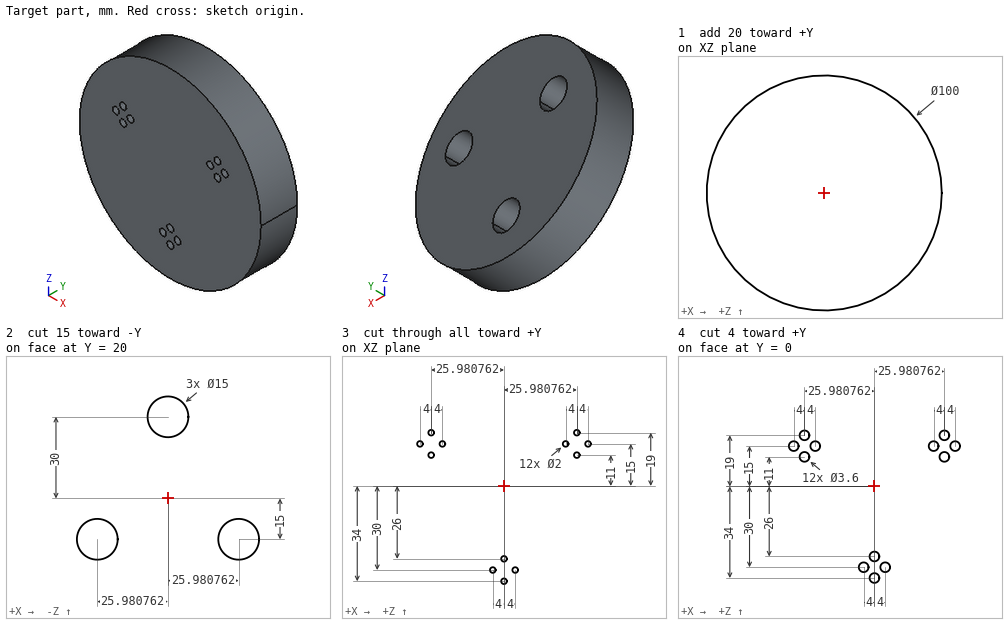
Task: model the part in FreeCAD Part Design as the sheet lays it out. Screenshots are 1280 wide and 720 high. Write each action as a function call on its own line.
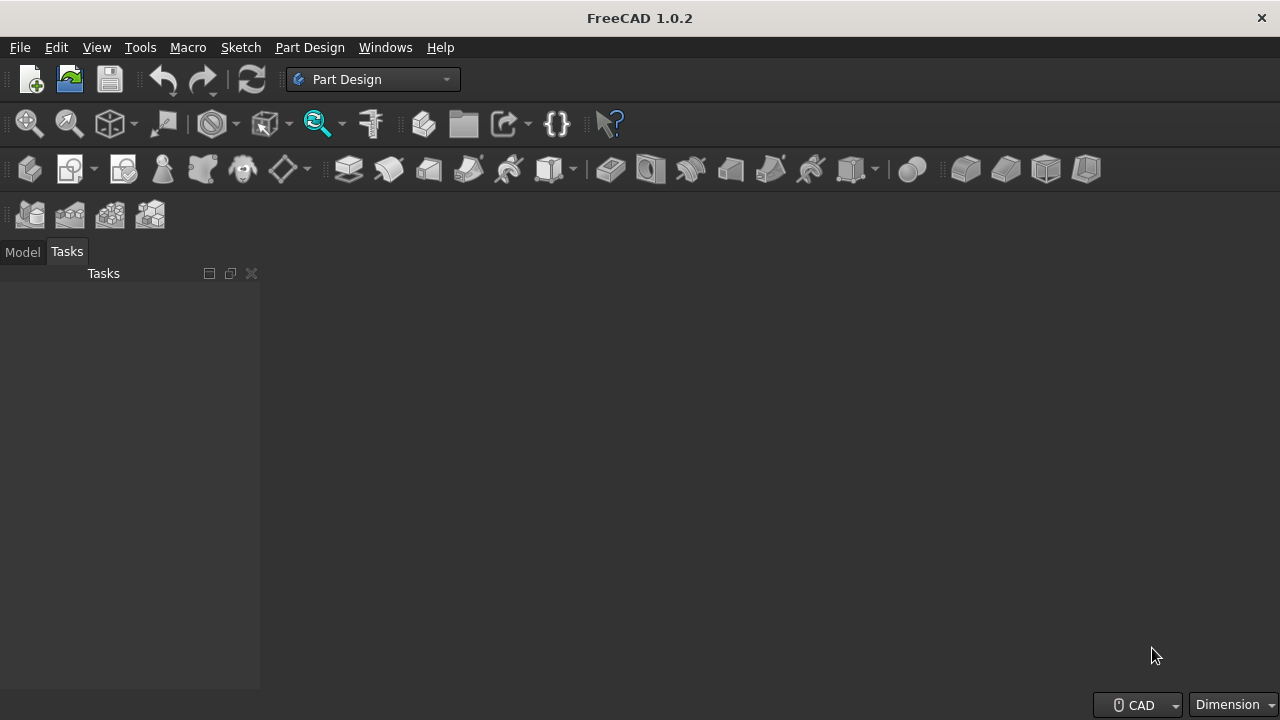
click(30, 80)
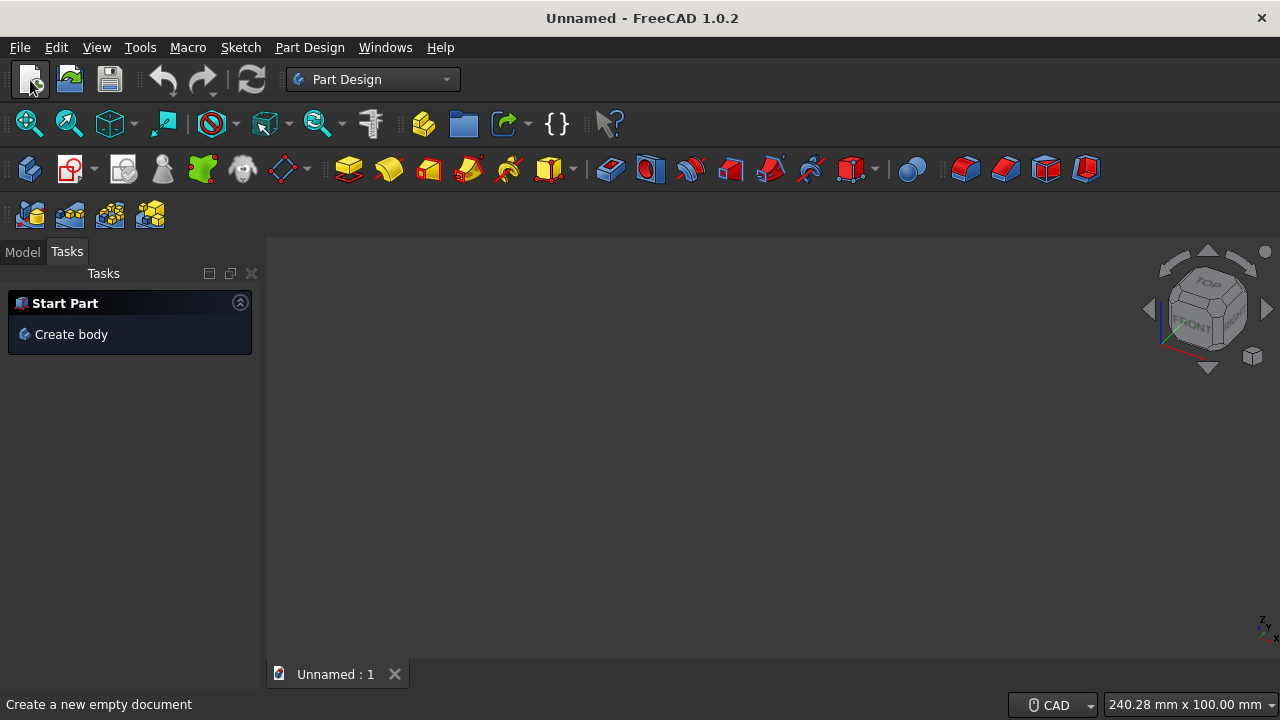
click(70, 170)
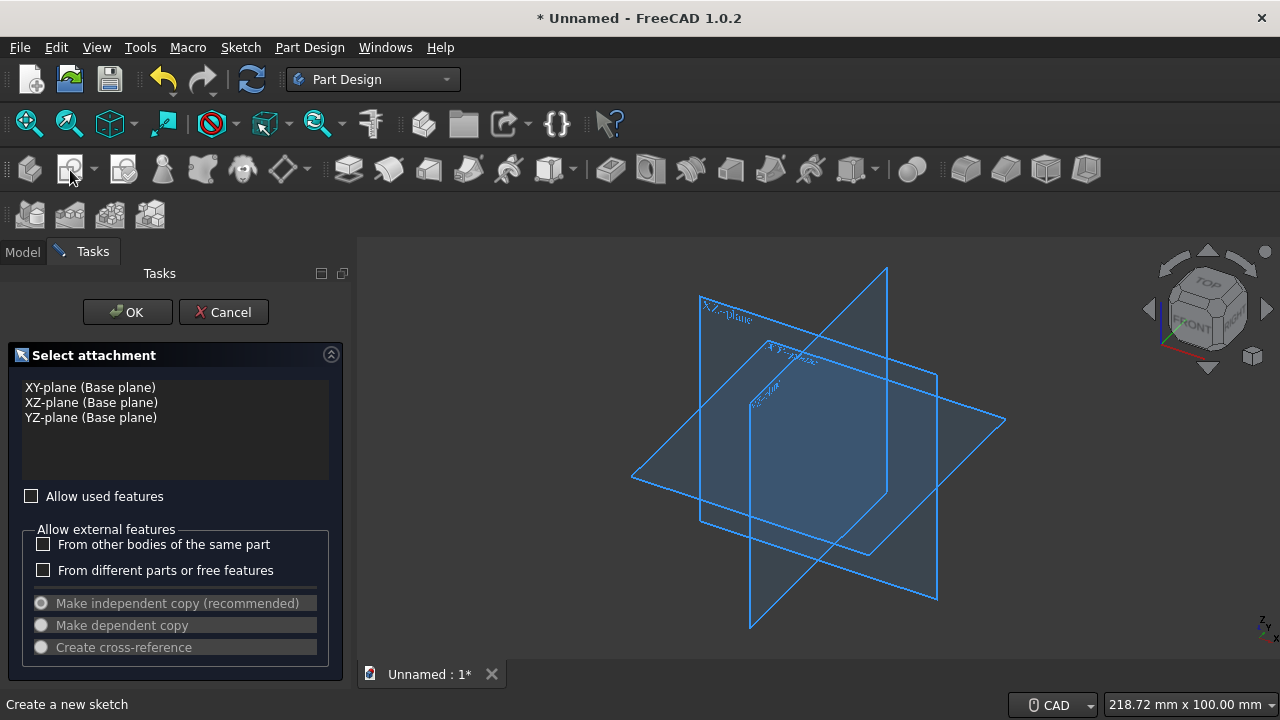
click(82, 402)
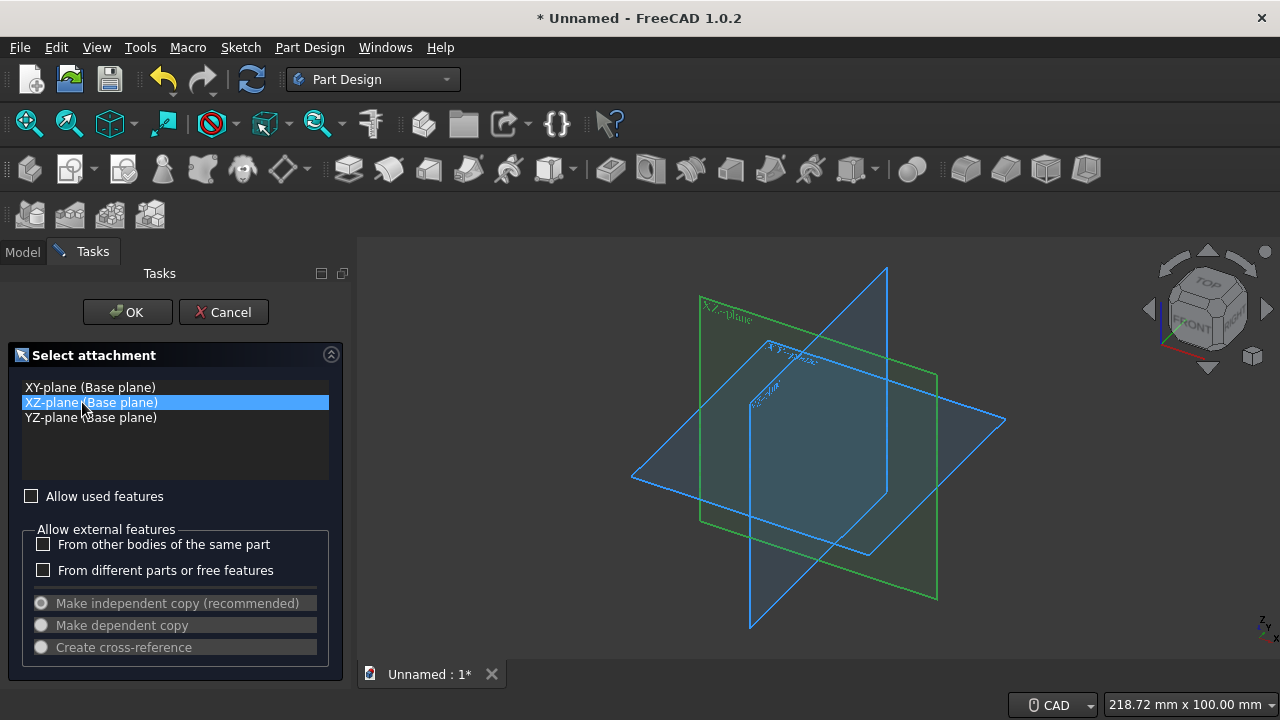
click(128, 312)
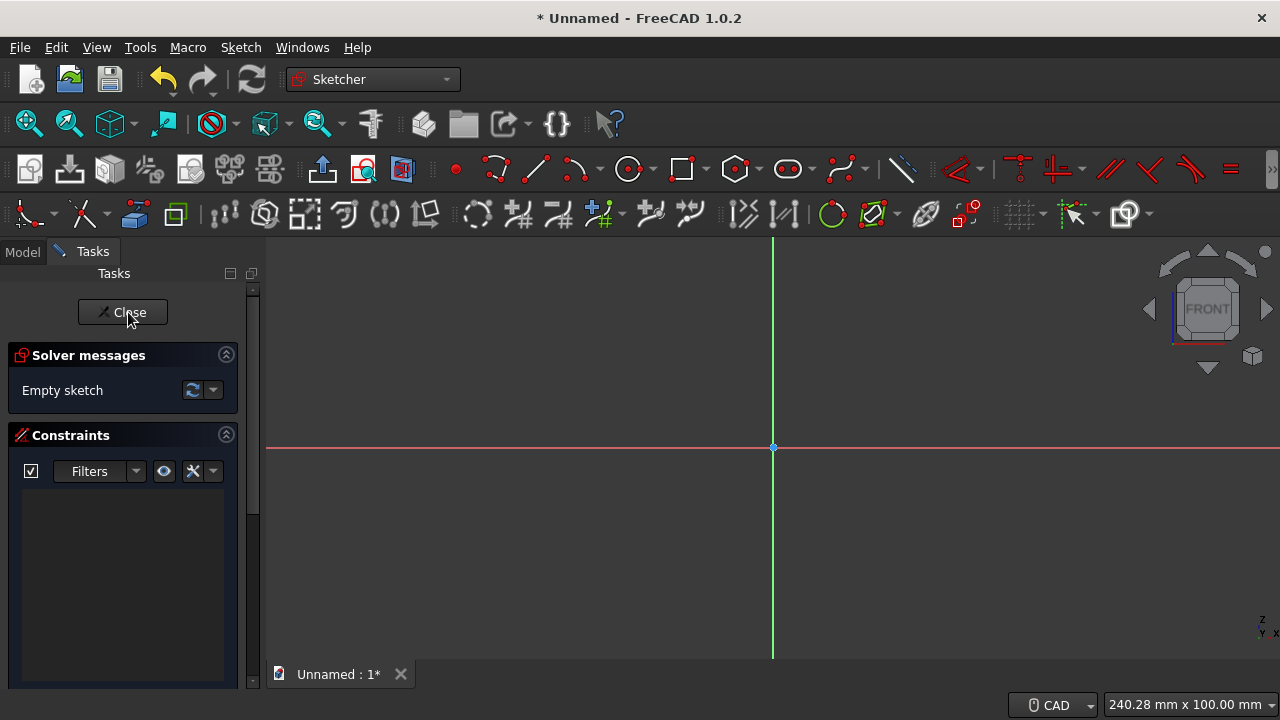
scroll(565, 448, down, 2)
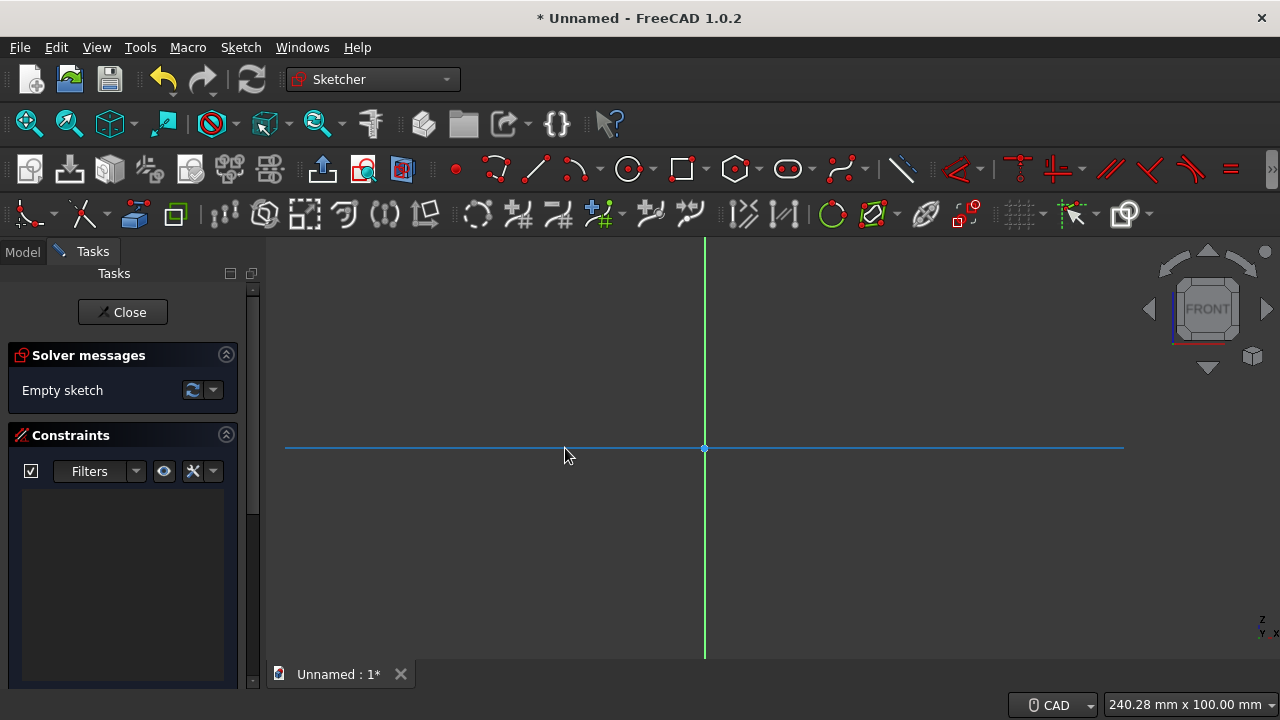
click(630, 170)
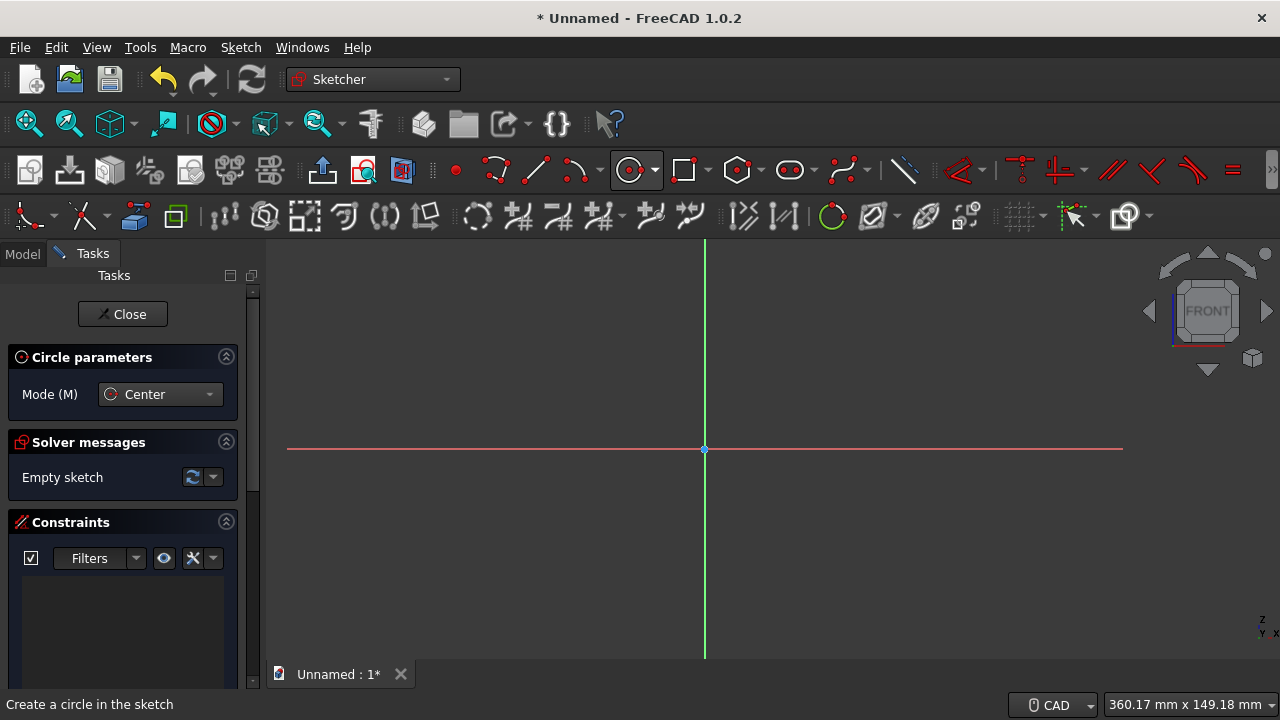
click(705, 449)
click(804, 350)
key(Escape)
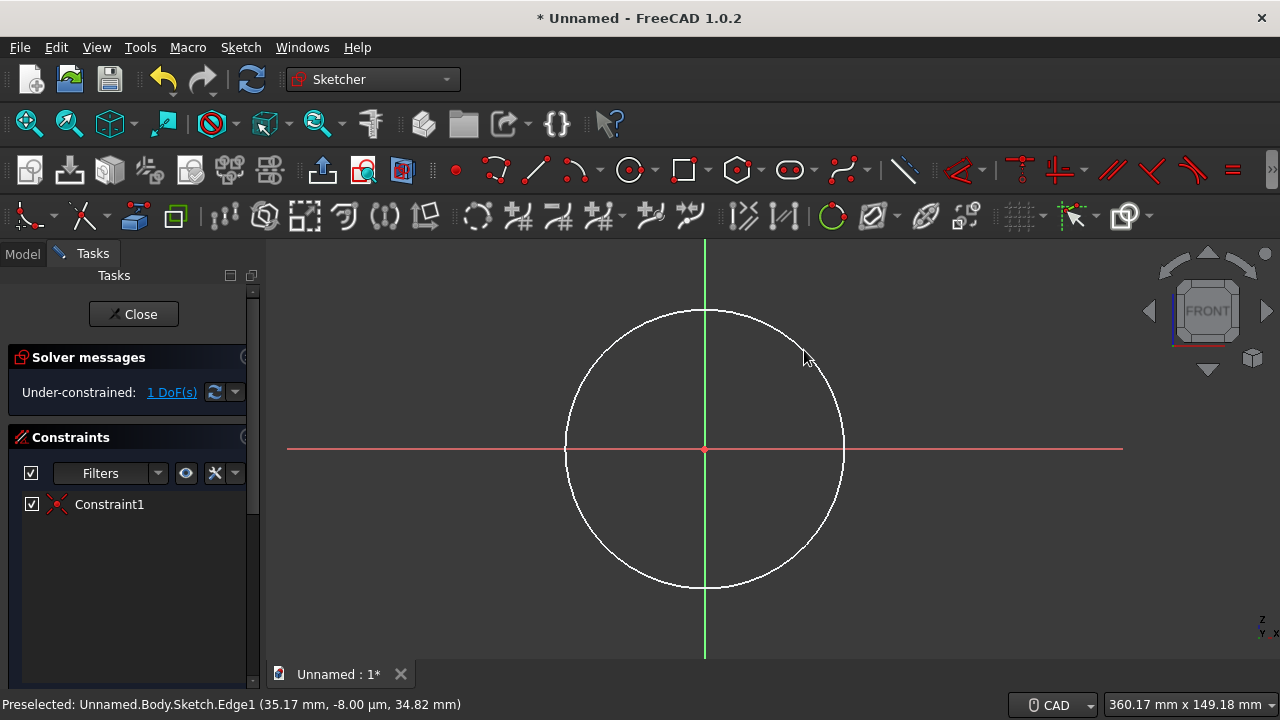
click(803, 350)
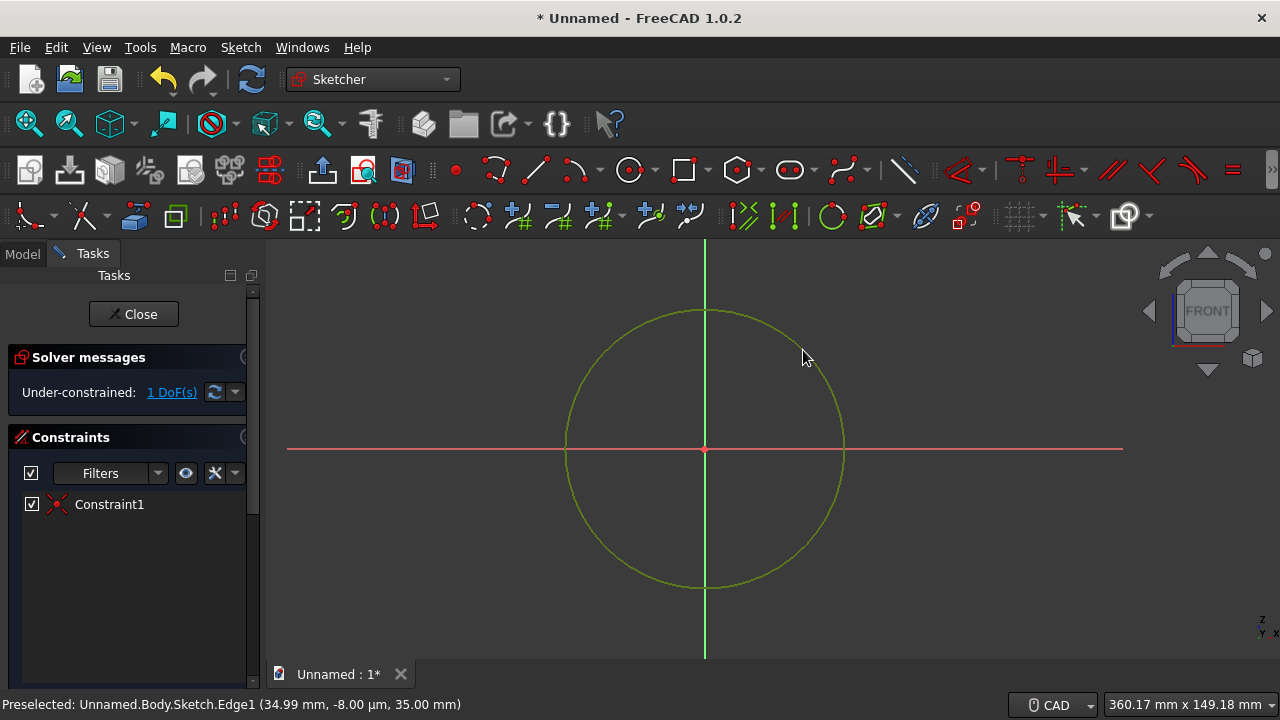
click(984, 170)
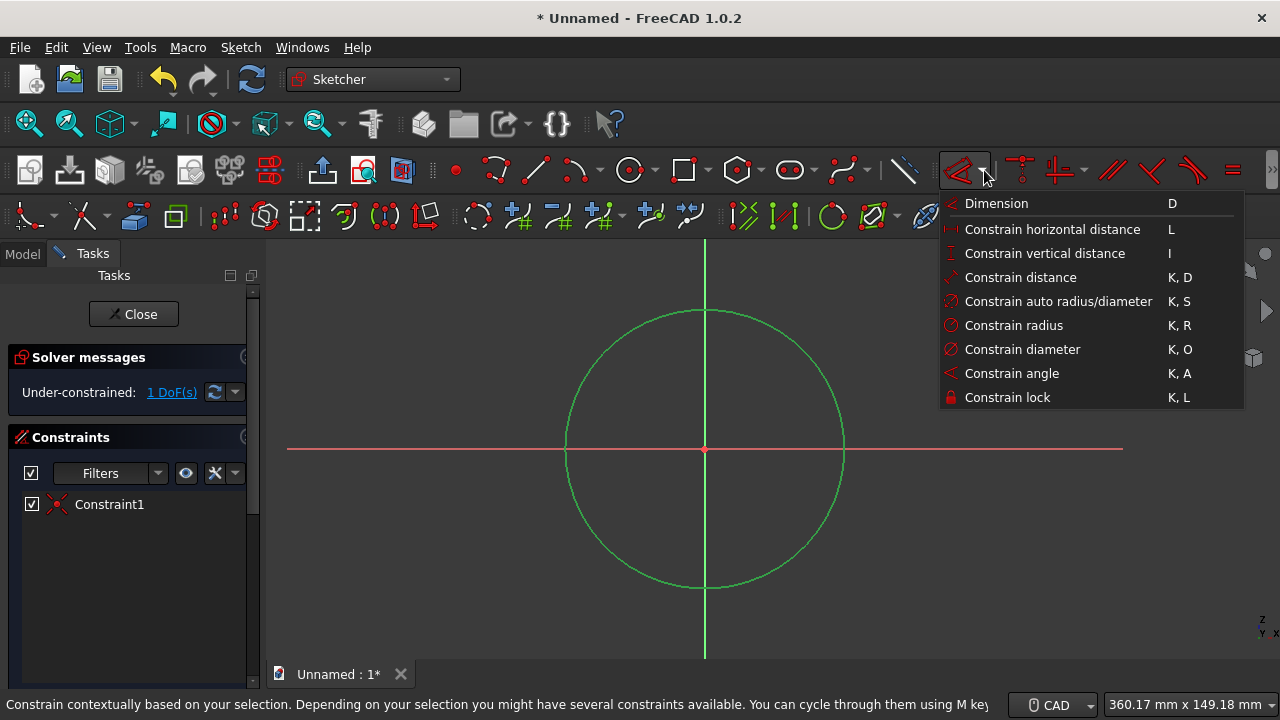
click(1092, 349)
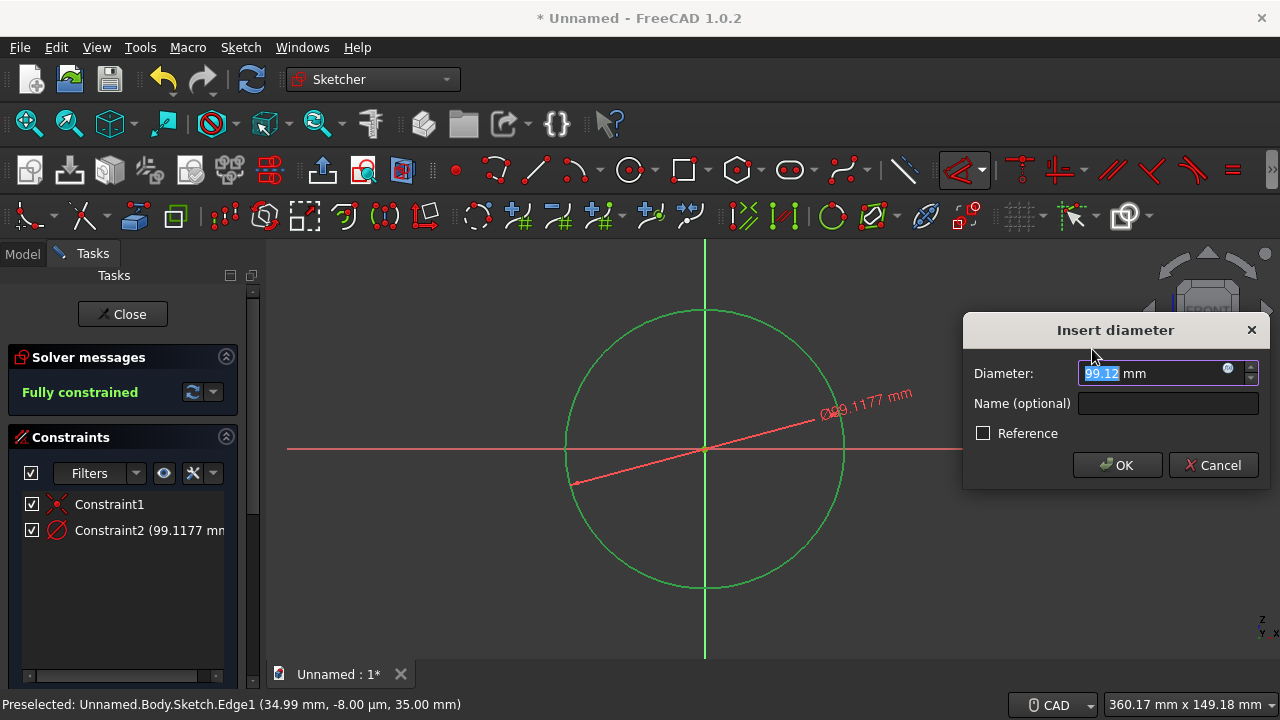
text(100)
key(Return)